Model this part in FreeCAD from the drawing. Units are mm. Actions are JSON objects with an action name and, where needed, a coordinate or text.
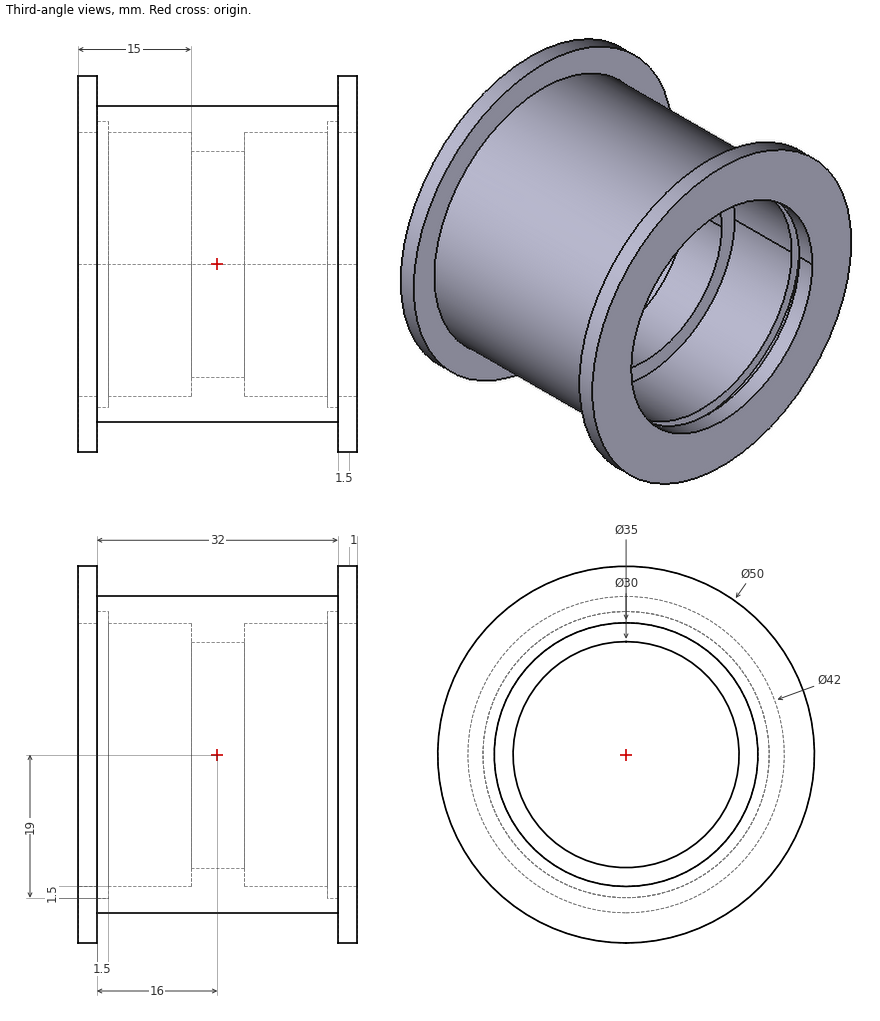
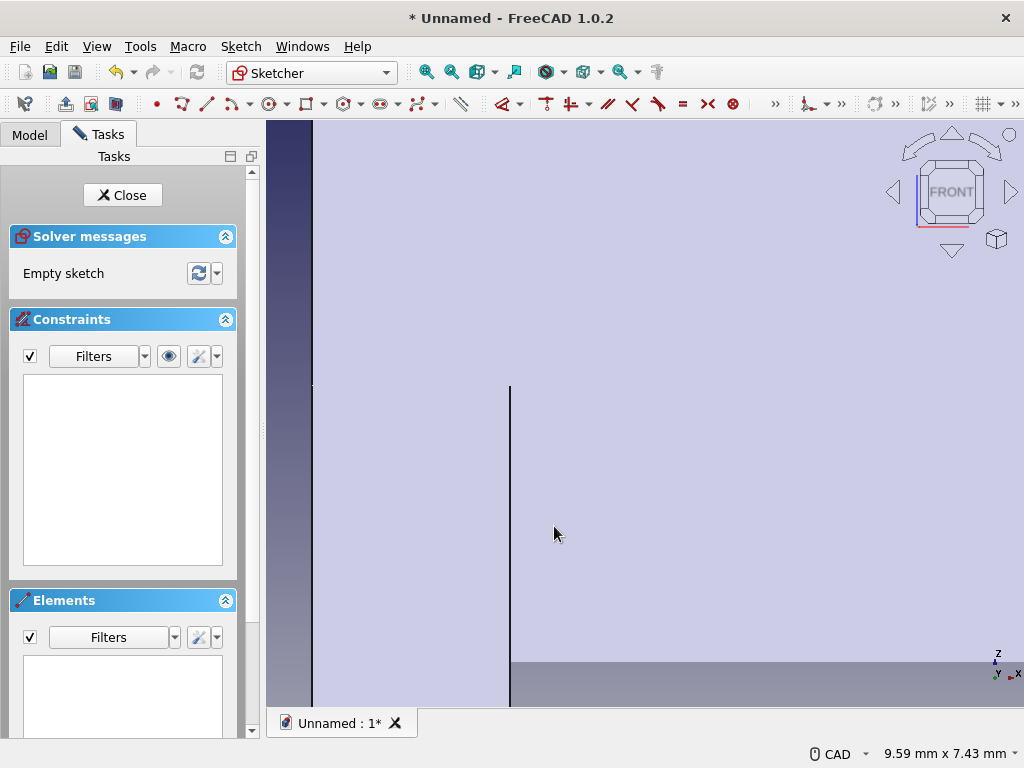
{"action": "scroll", "coordinate": [577, 398], "scroll_direction": "up", "scroll_amount": 4}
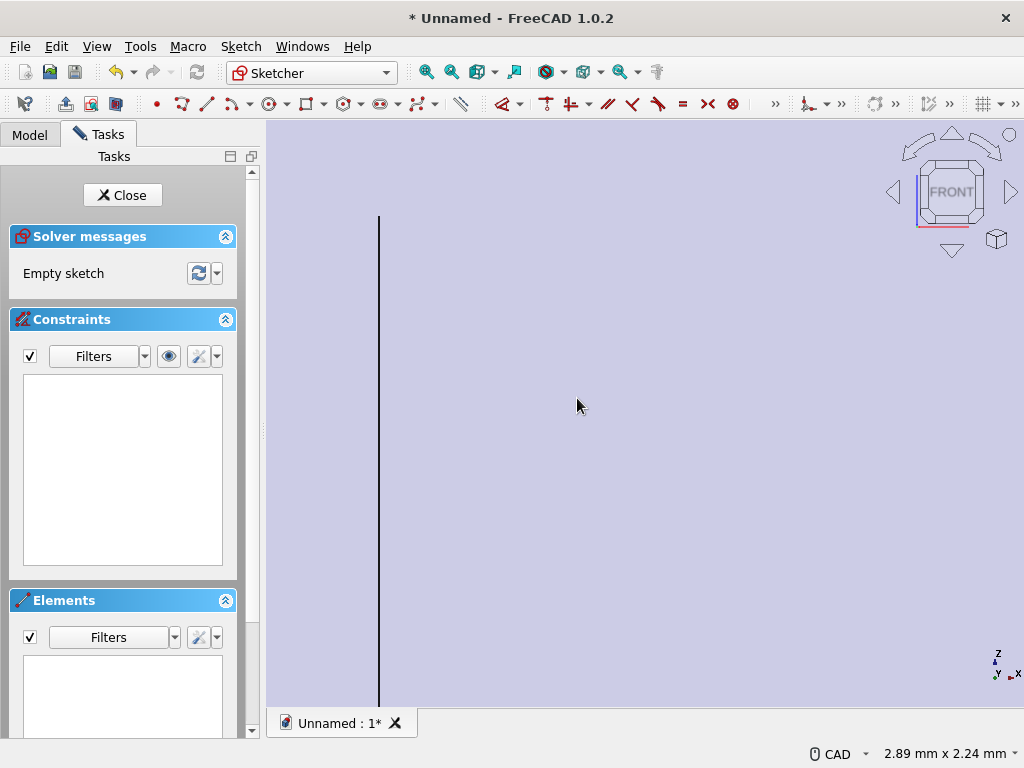
{"action": "key", "text": "g r"}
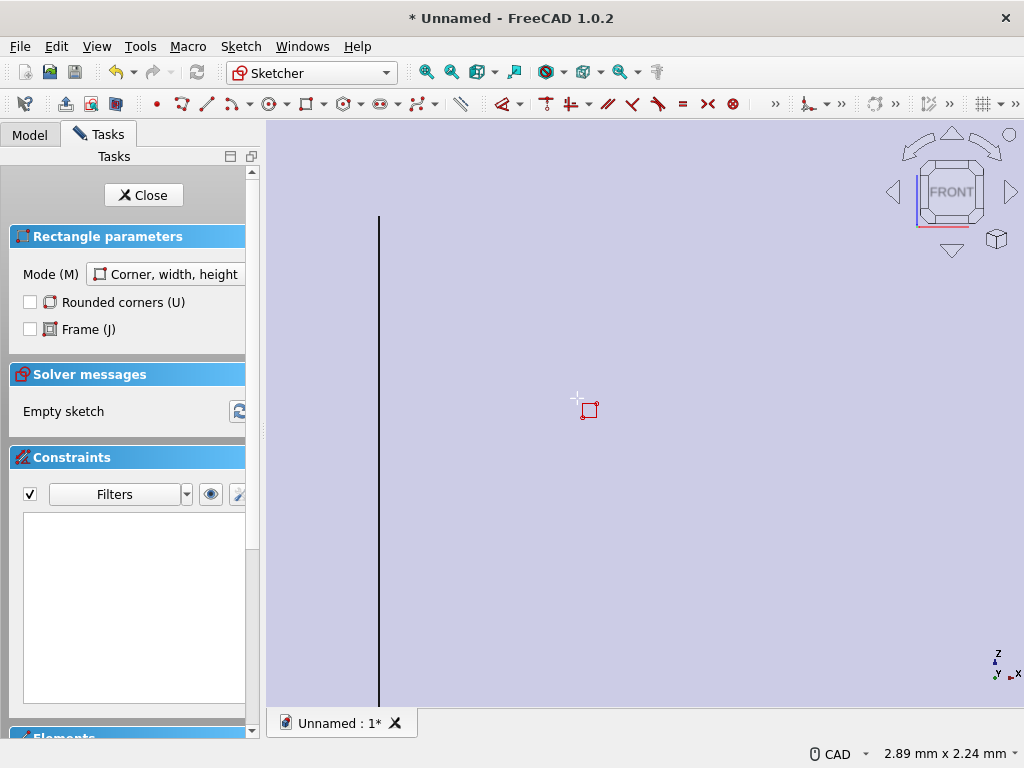
{"action": "left_click", "coordinate": [379, 216]}
{"action": "mouse_move", "coordinate": [772, 610]}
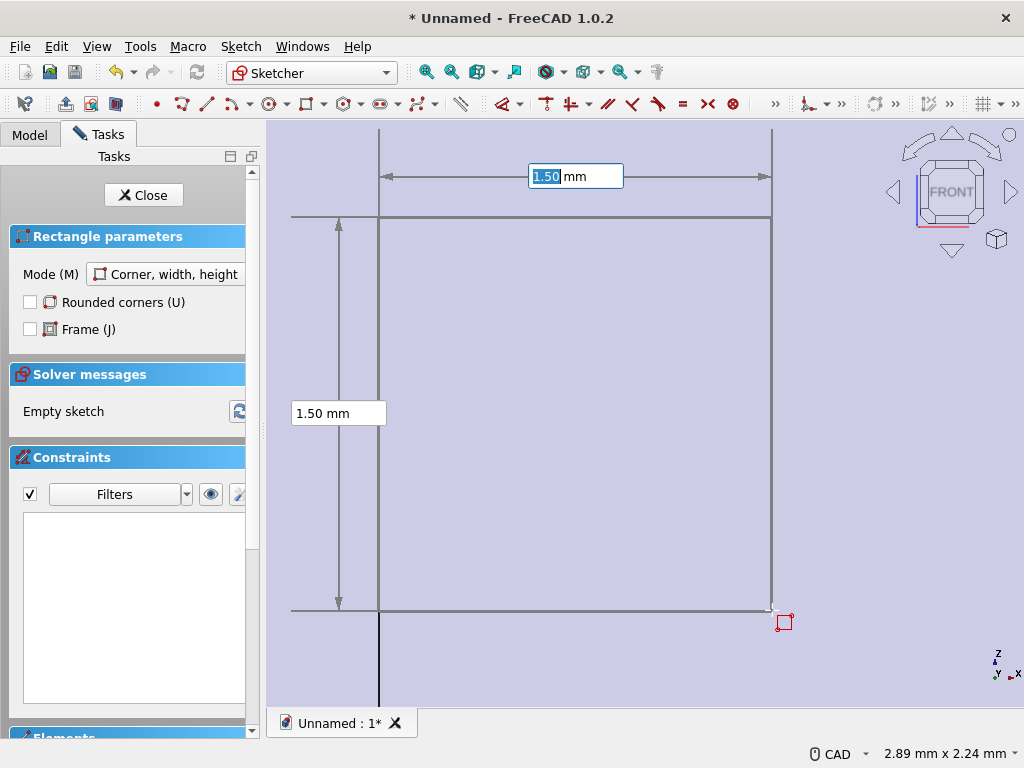
{"action": "type", "text": "1.5"}
{"action": "key", "text": "Tab"}
{"action": "type", "text": "1.5"}
{"action": "key", "text": "Return"}
{"action": "key", "text": "Escape"}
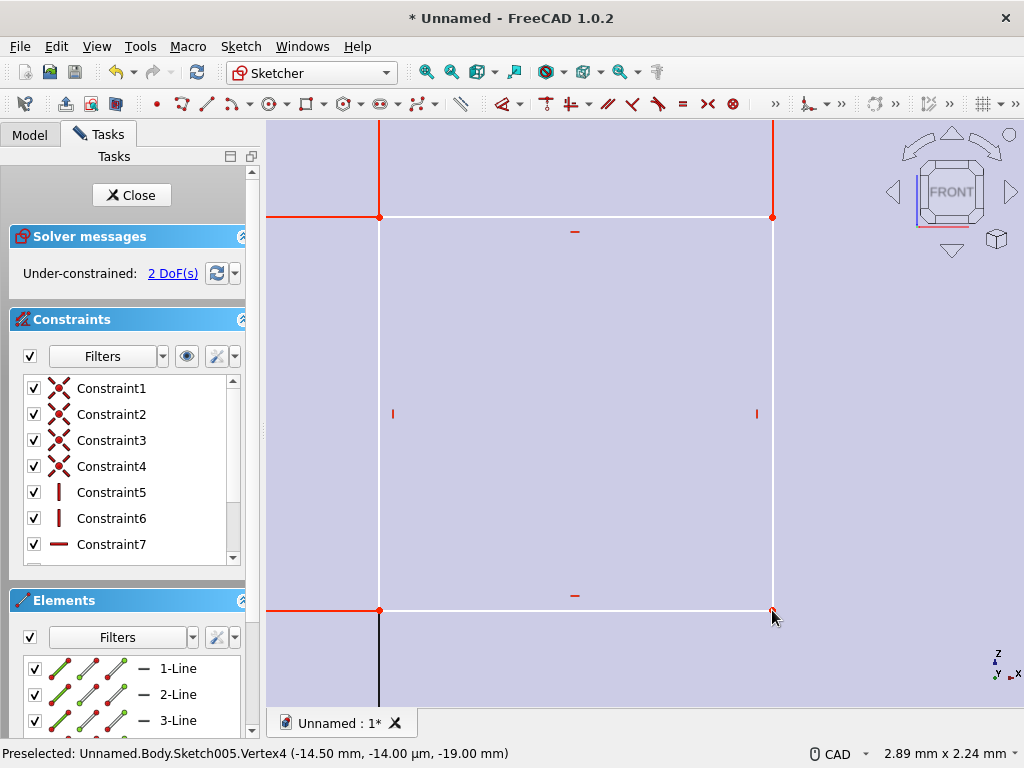
{"action": "left_click", "coordinate": [502, 104]}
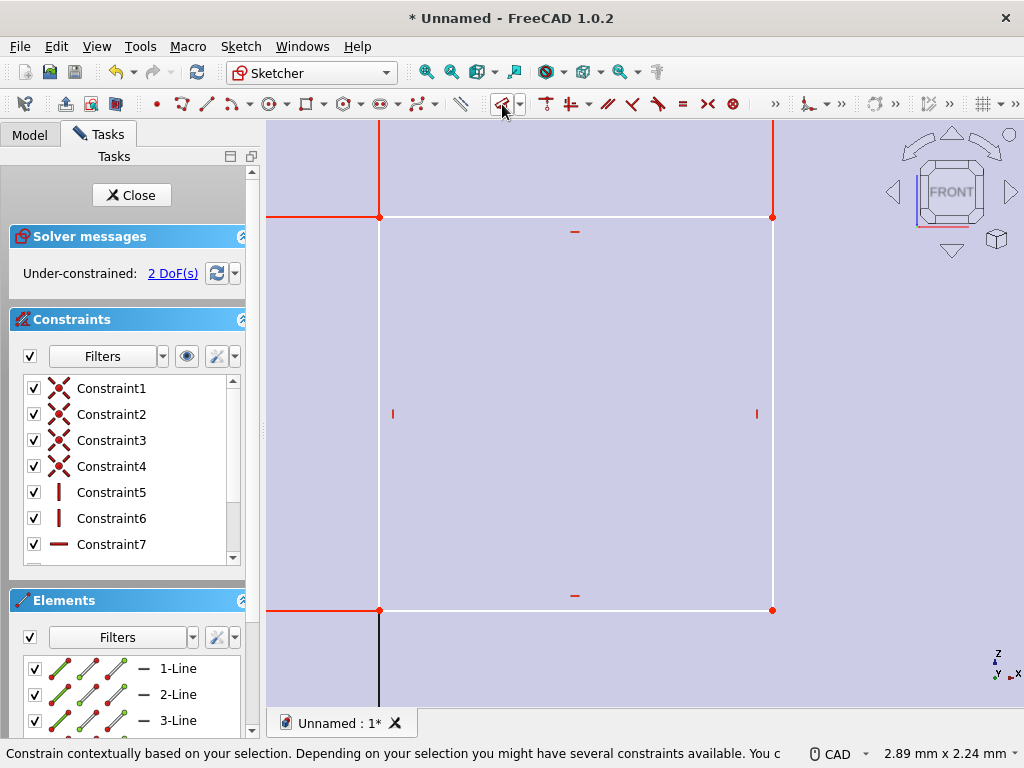
{"action": "left_click", "coordinate": [379, 217]}
{"action": "left_click", "coordinate": [619, 251]}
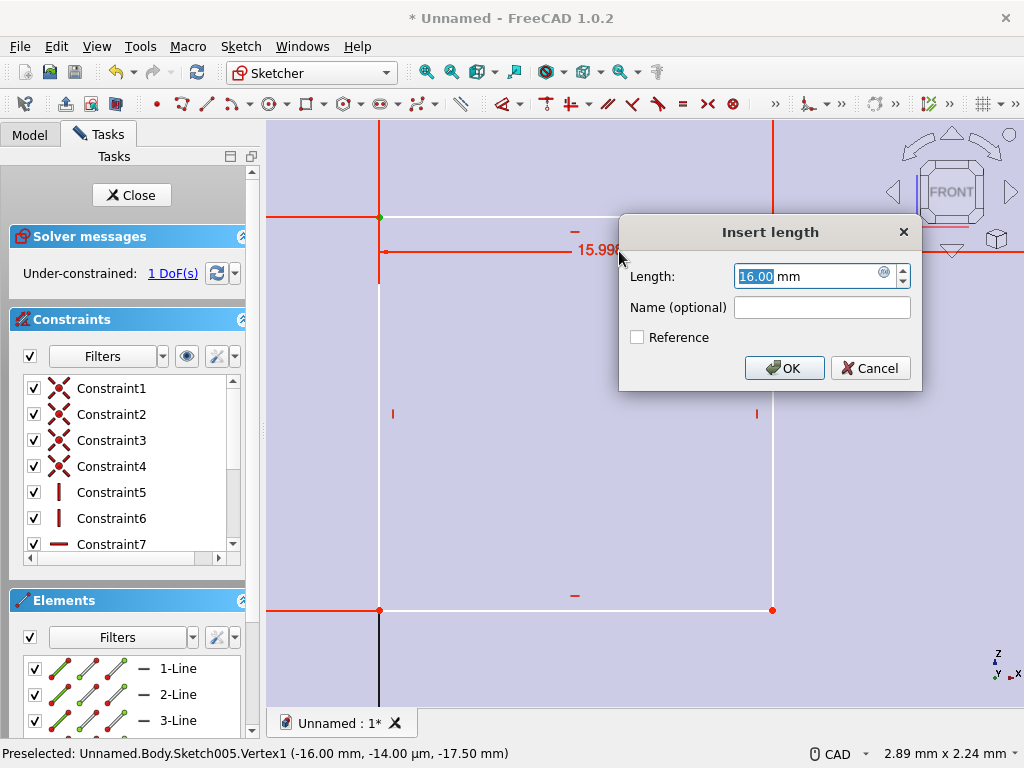
{"action": "type", "text": "16"}
{"action": "key", "text": "Return"}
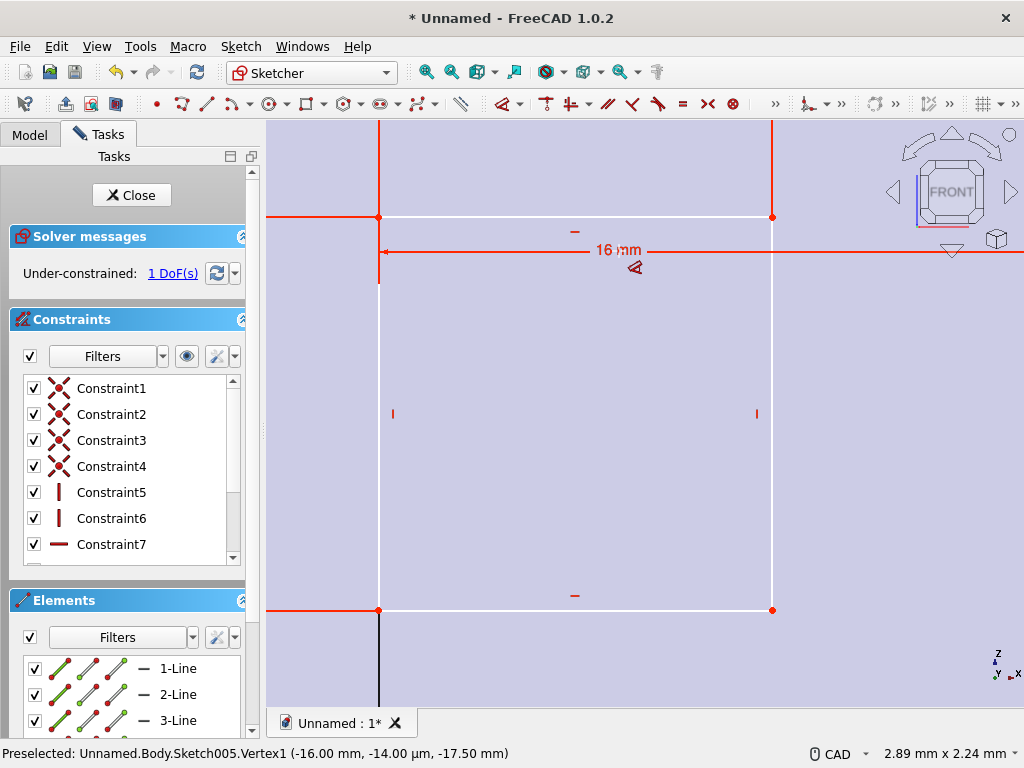
{"action": "left_click", "coordinate": [379, 611]}
{"action": "left_click", "coordinate": [345, 379]}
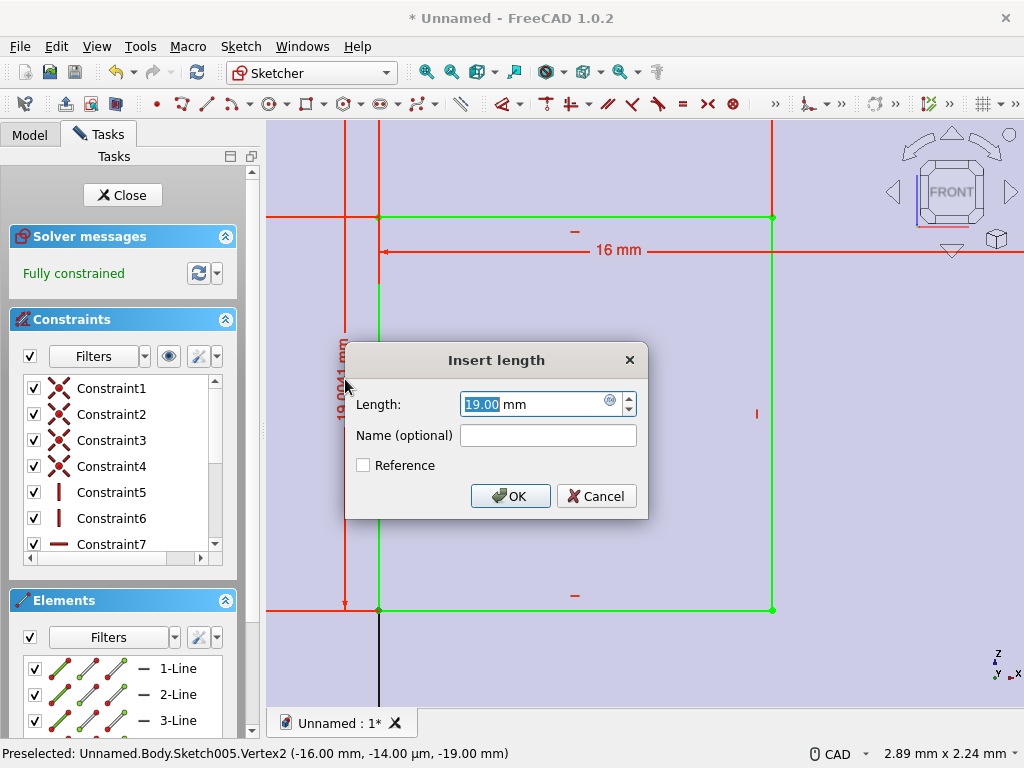
{"action": "type", "text": "19"}
{"action": "key", "text": "Return"}
{"action": "key", "text": "Escape"}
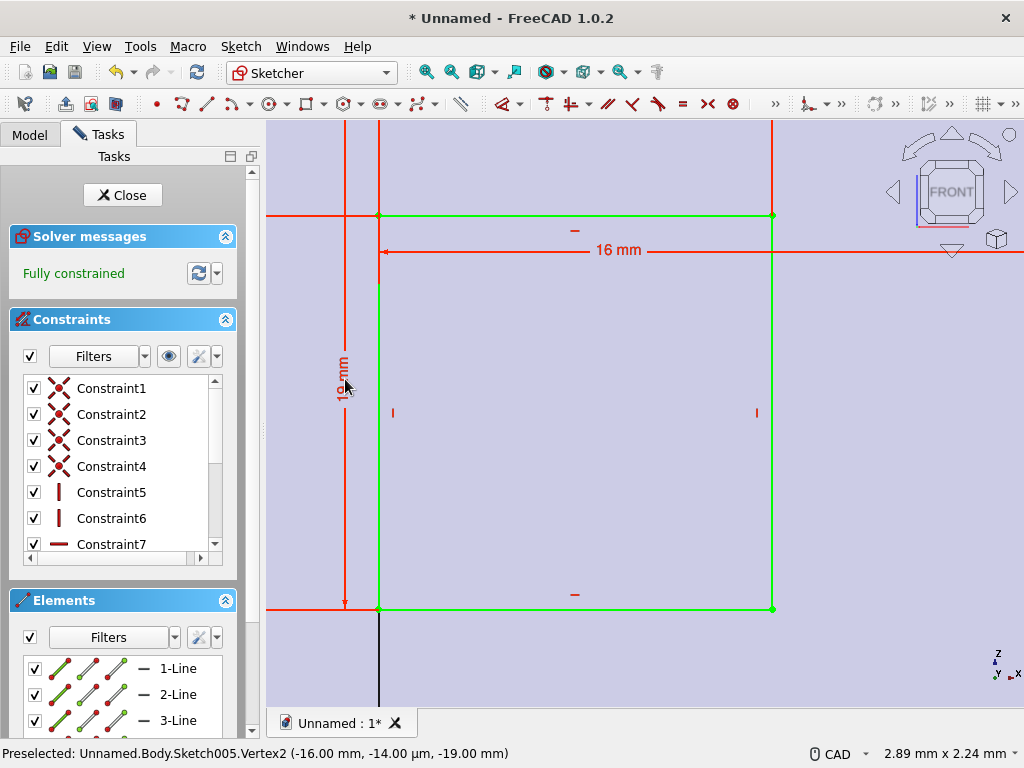
{"action": "left_click", "coordinate": [123, 195]}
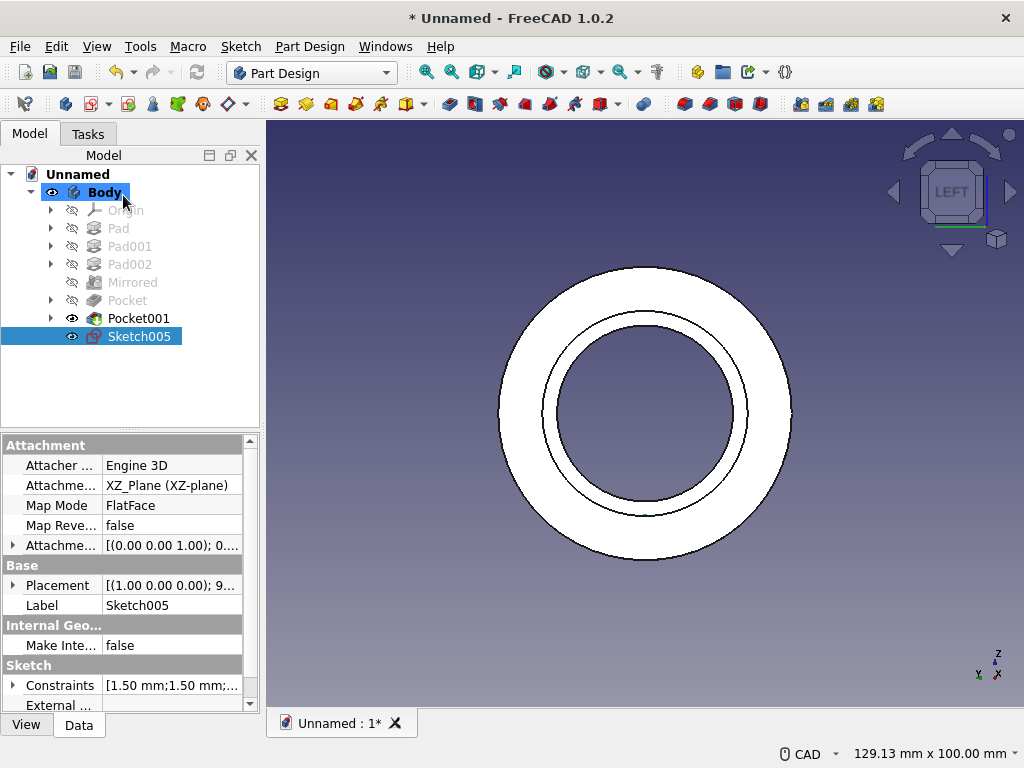
{"action": "left_click", "coordinate": [500, 104]}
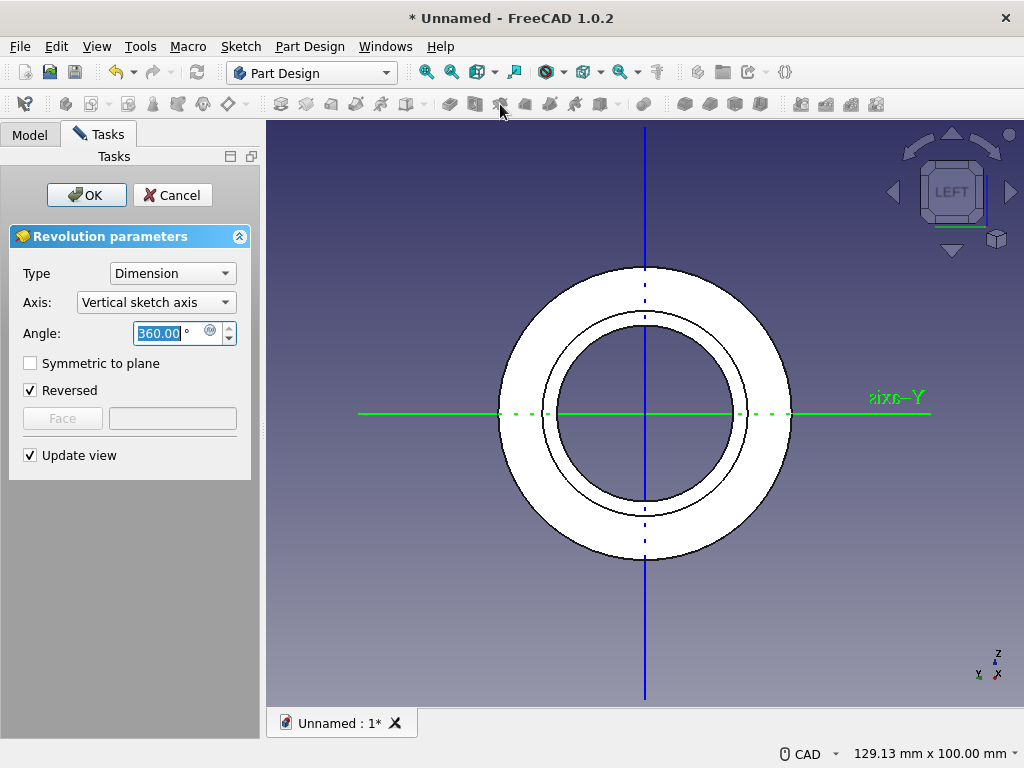
{"action": "left_click", "coordinate": [157, 302]}